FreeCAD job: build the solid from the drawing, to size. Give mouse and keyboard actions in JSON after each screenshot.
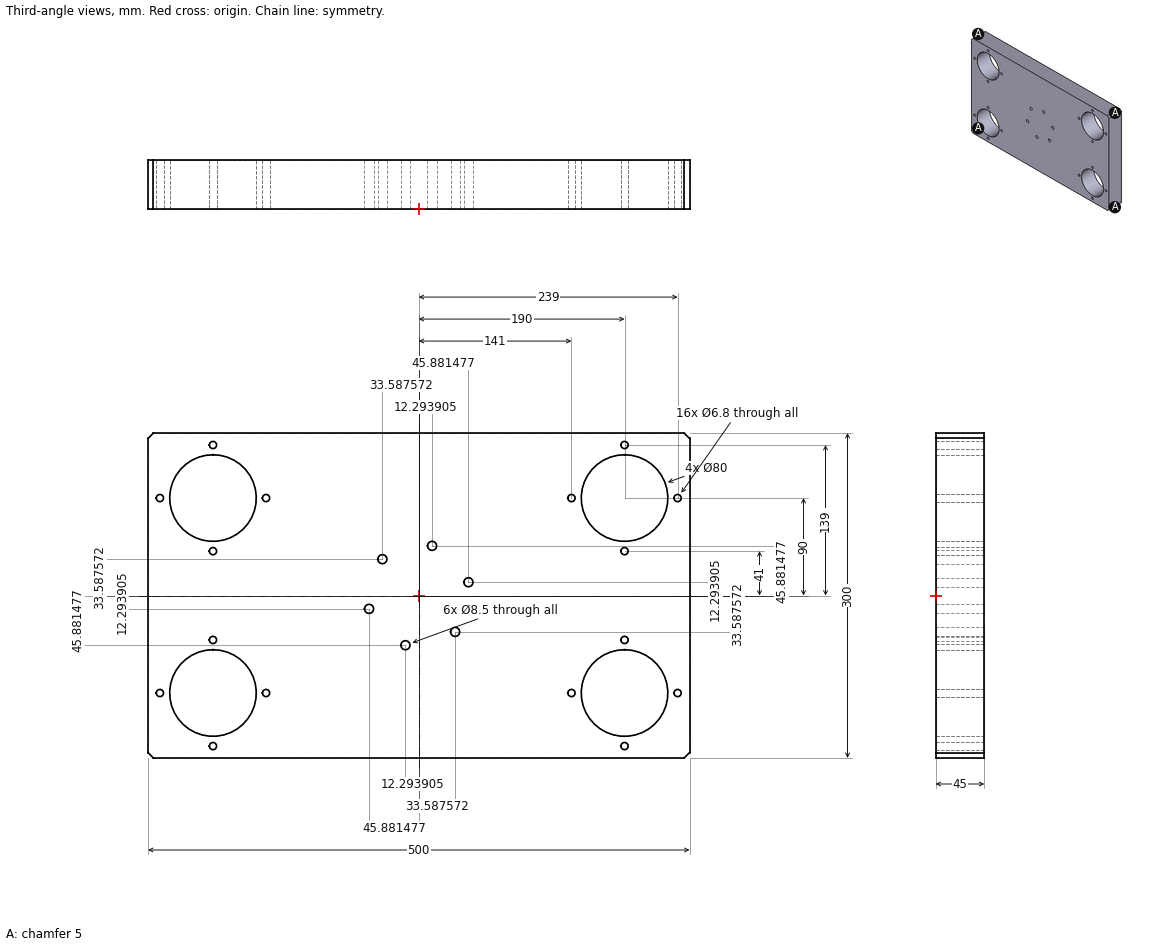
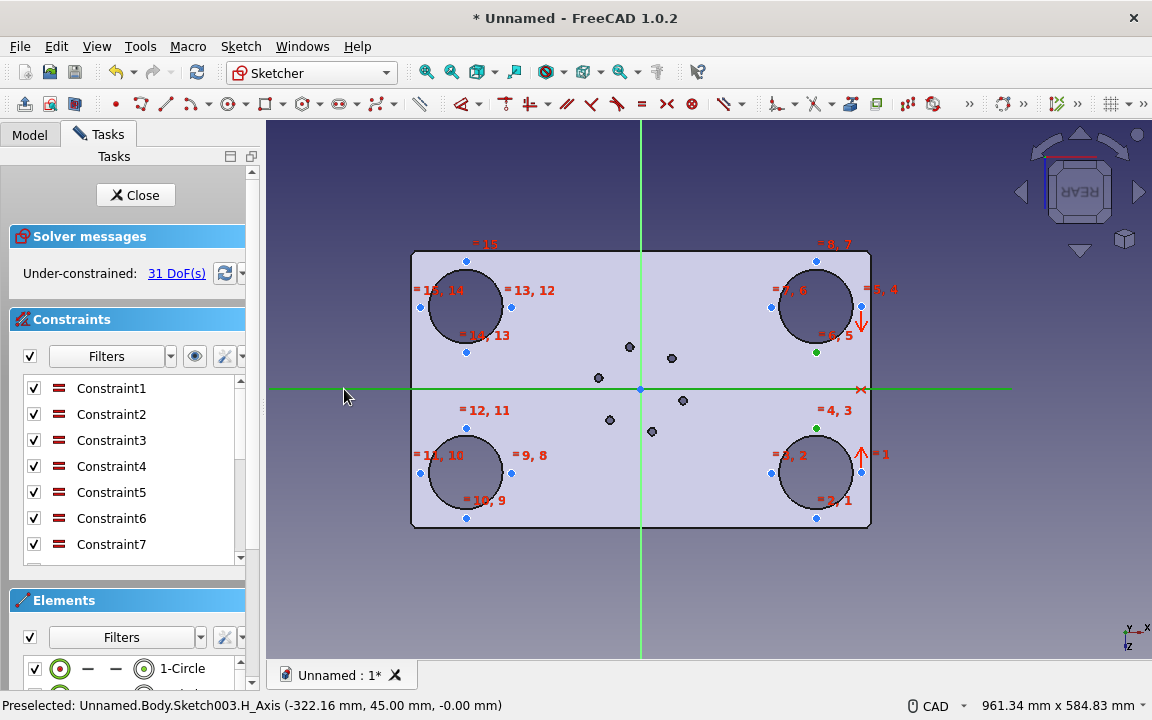
{"action": "left_click", "coordinate": [667, 104]}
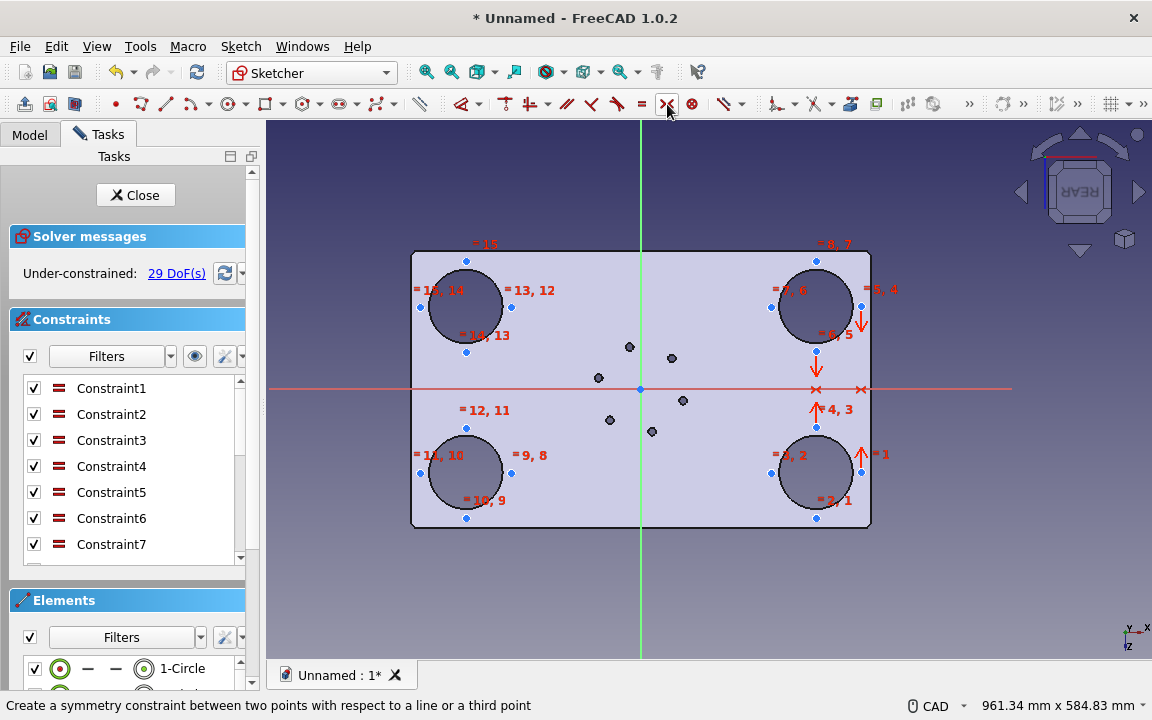
{"action": "left_click", "coordinate": [771, 473]}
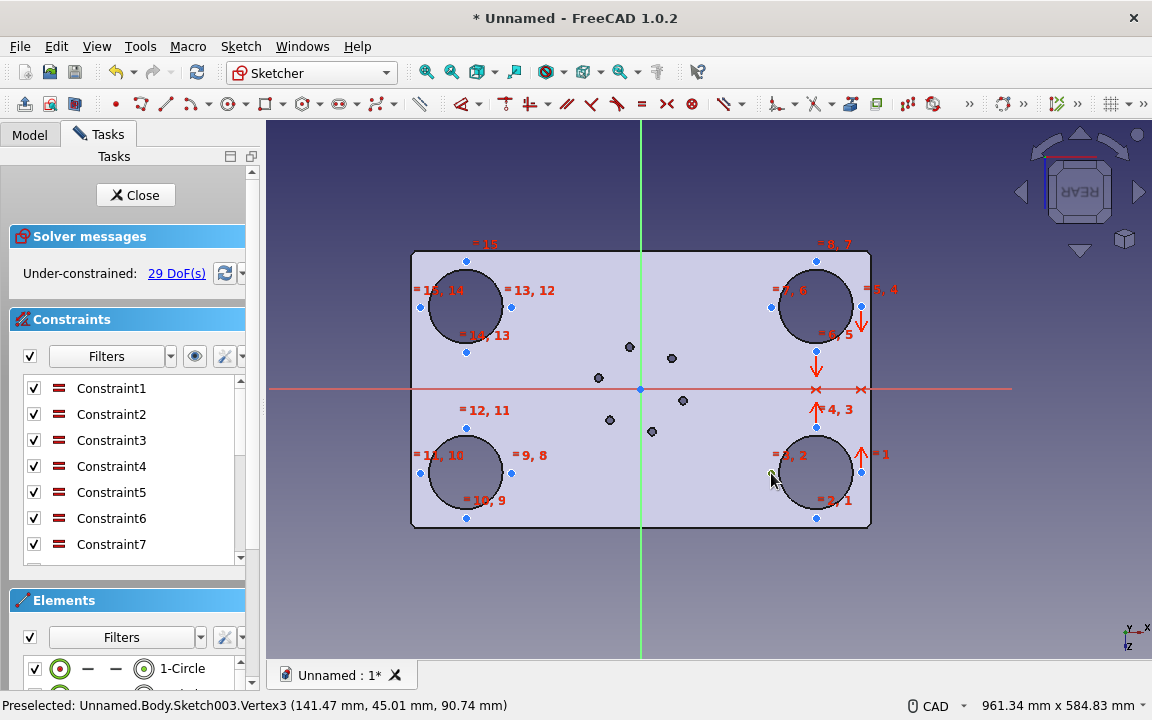
{"action": "left_click", "coordinate": [771, 308]}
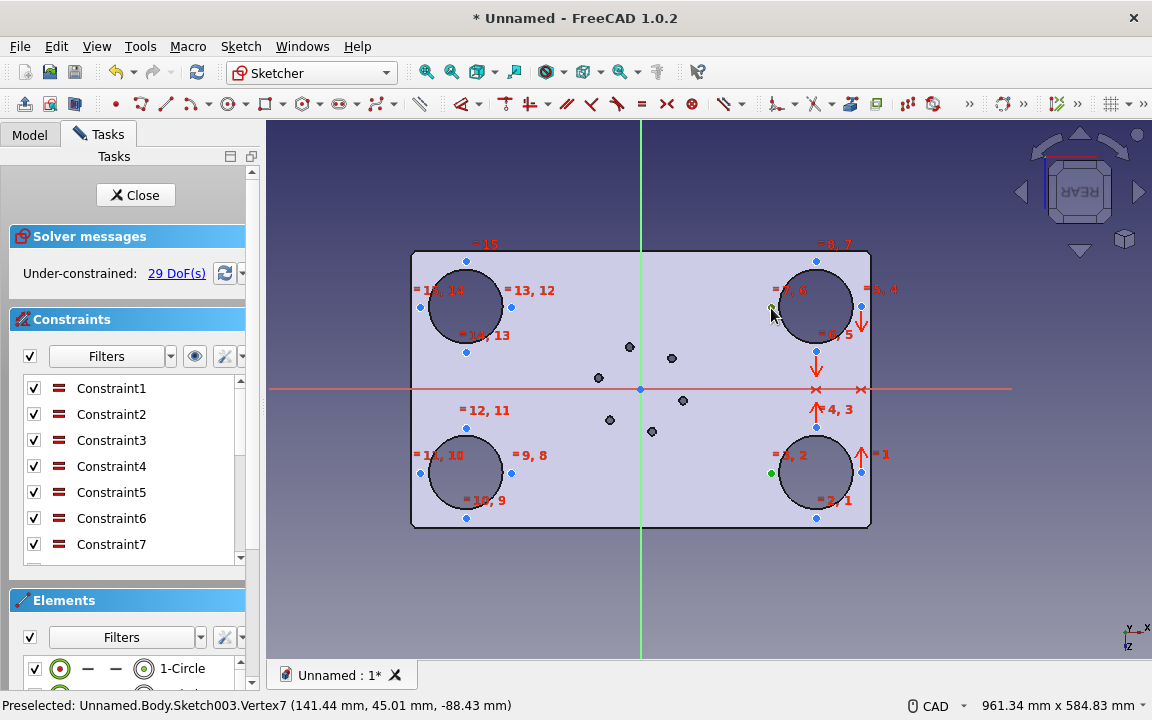
{"action": "left_click", "coordinate": [344, 389]}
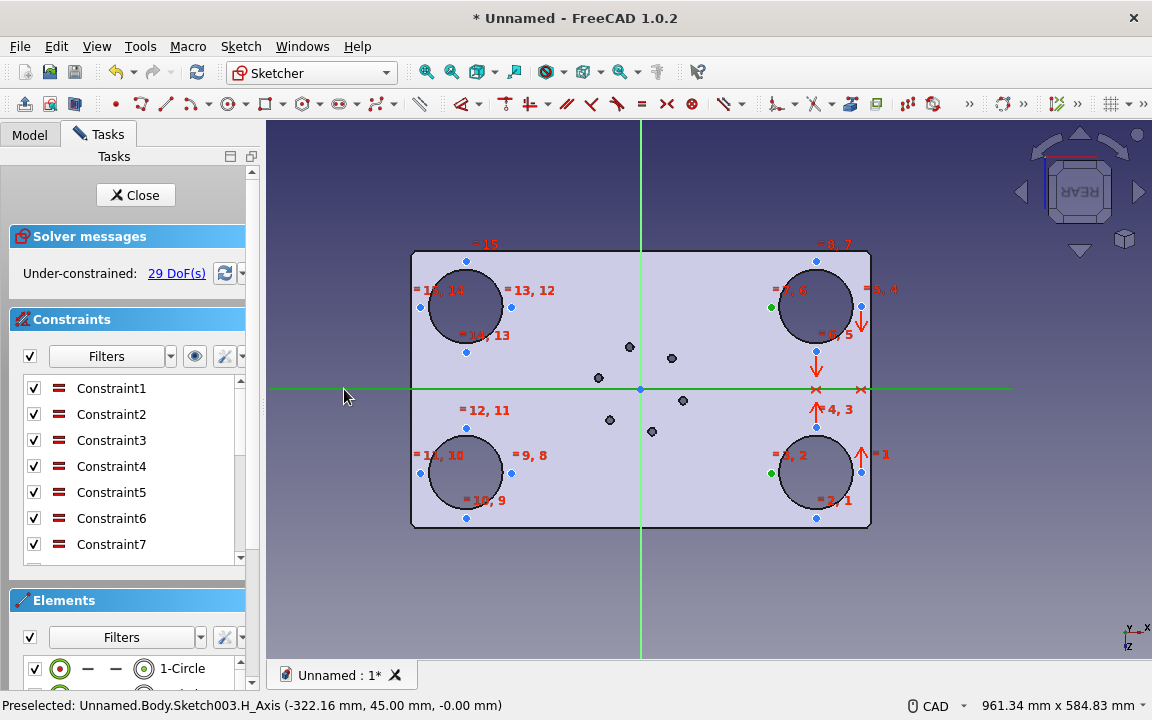
{"action": "left_click", "coordinate": [667, 104]}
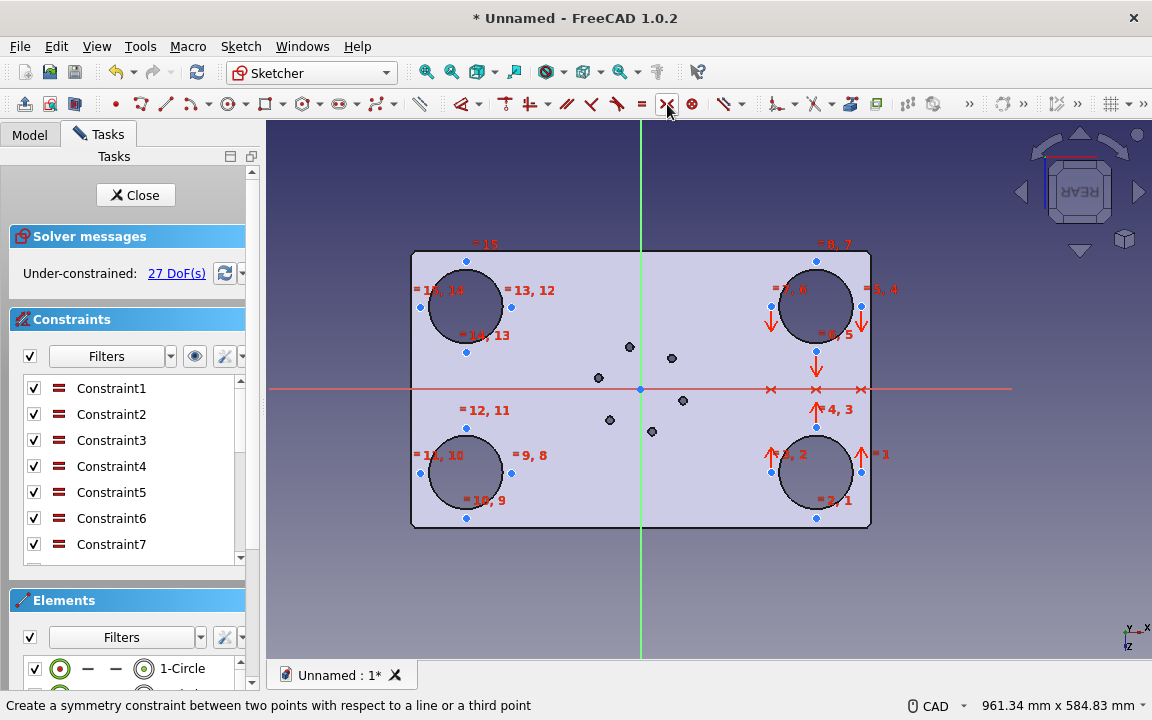
{"action": "left_click", "coordinate": [816, 518]}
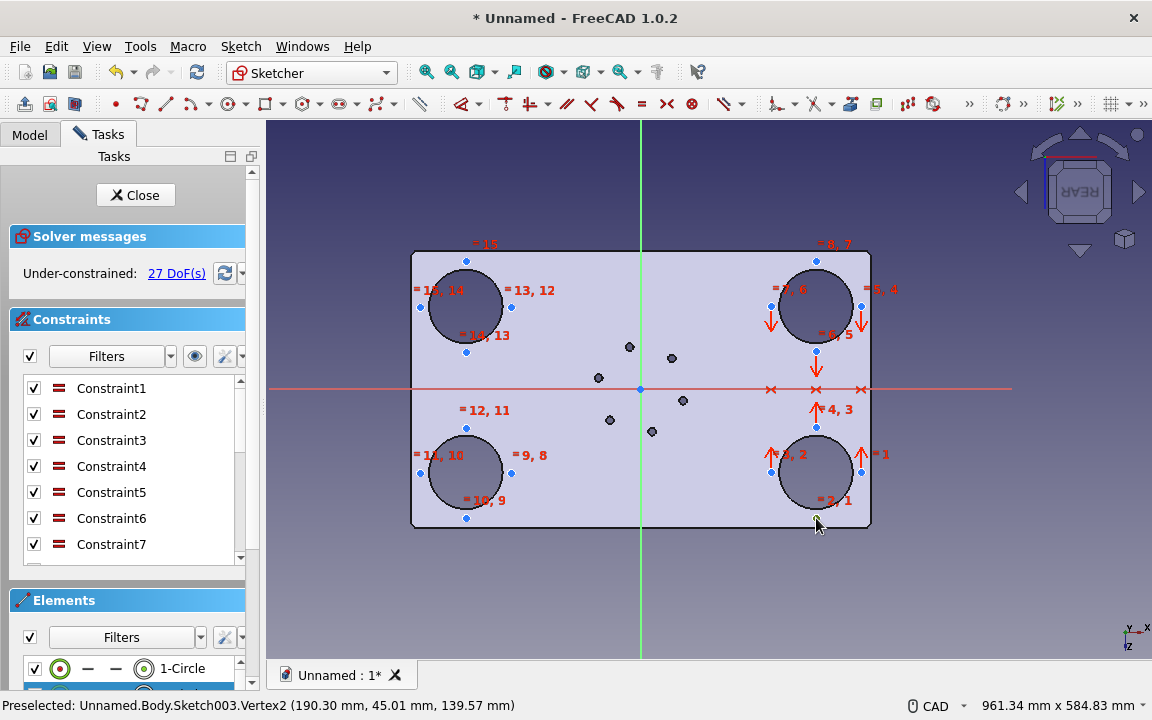
{"action": "left_click", "coordinate": [816, 262]}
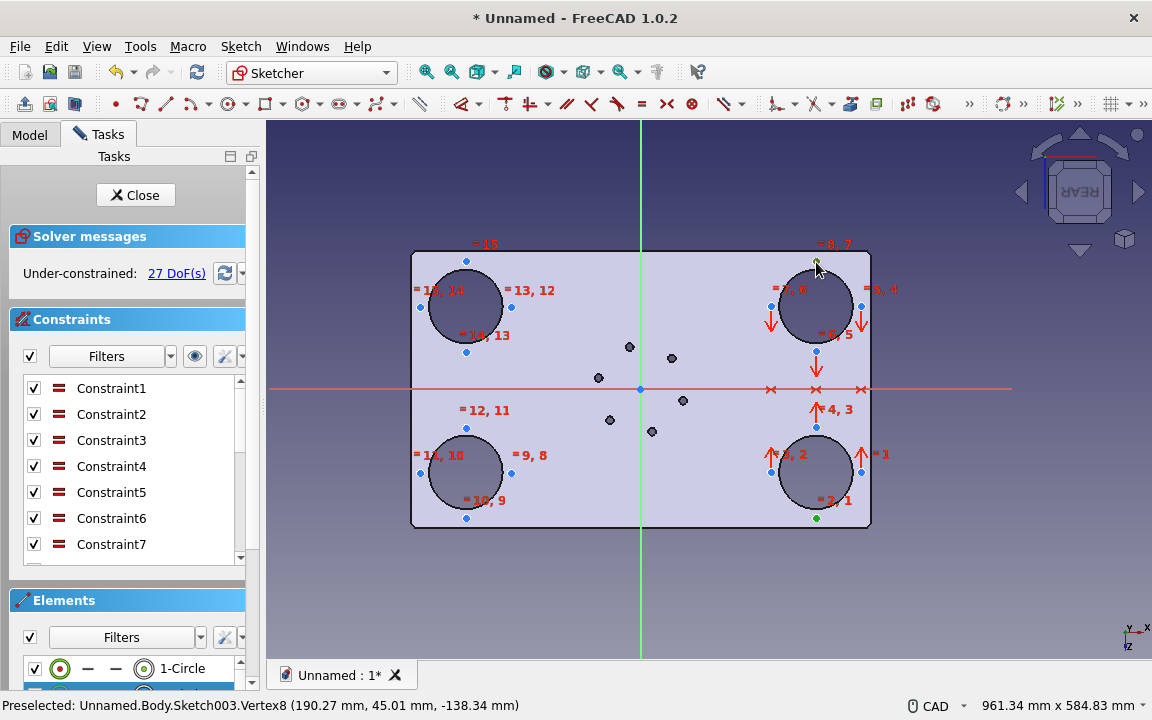
{"action": "left_click", "coordinate": [344, 389]}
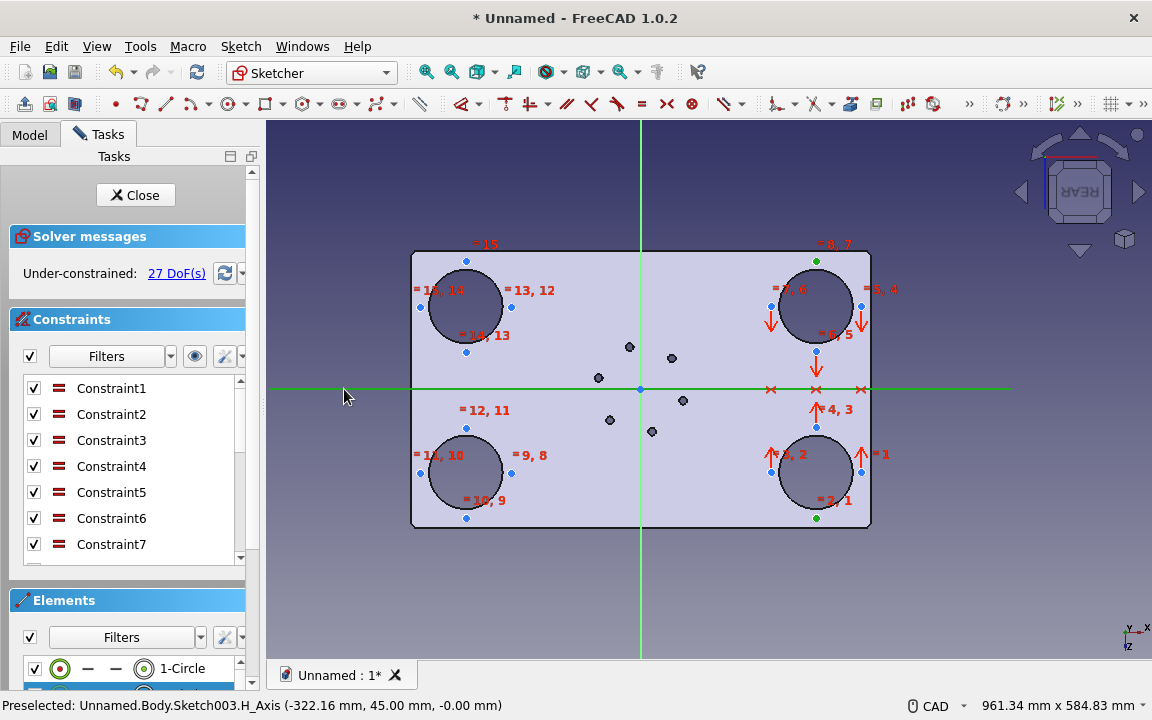
{"action": "left_click", "coordinate": [667, 104]}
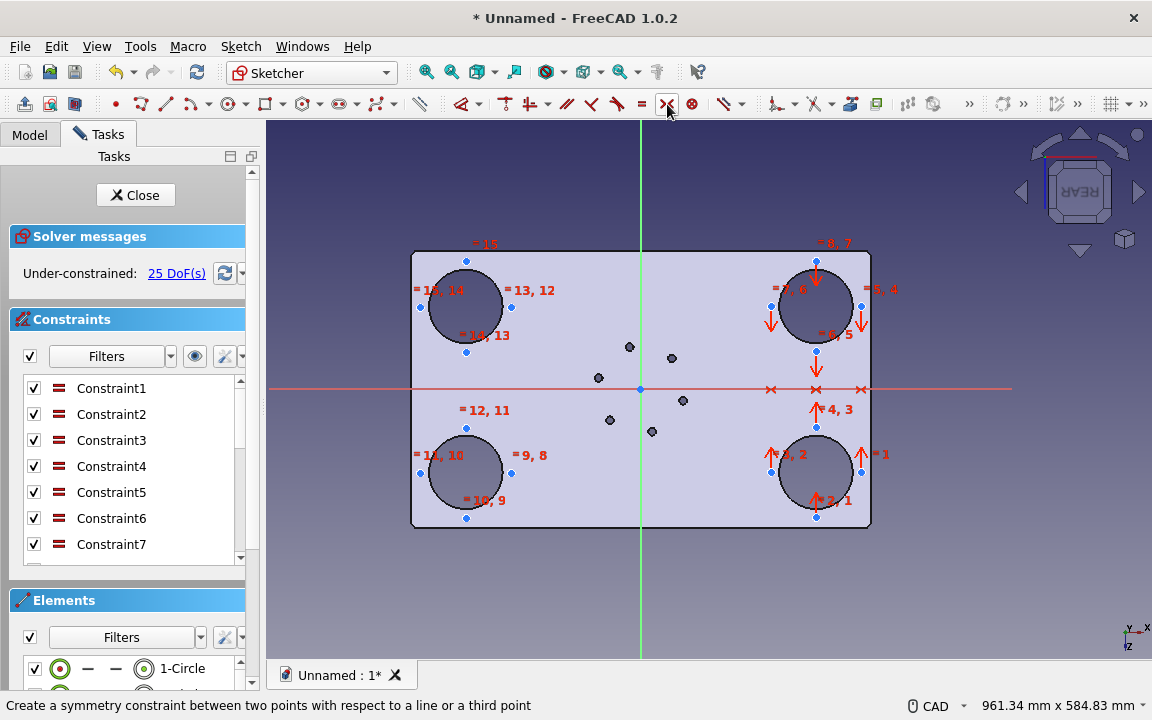
{"action": "left_click", "coordinate": [771, 472]}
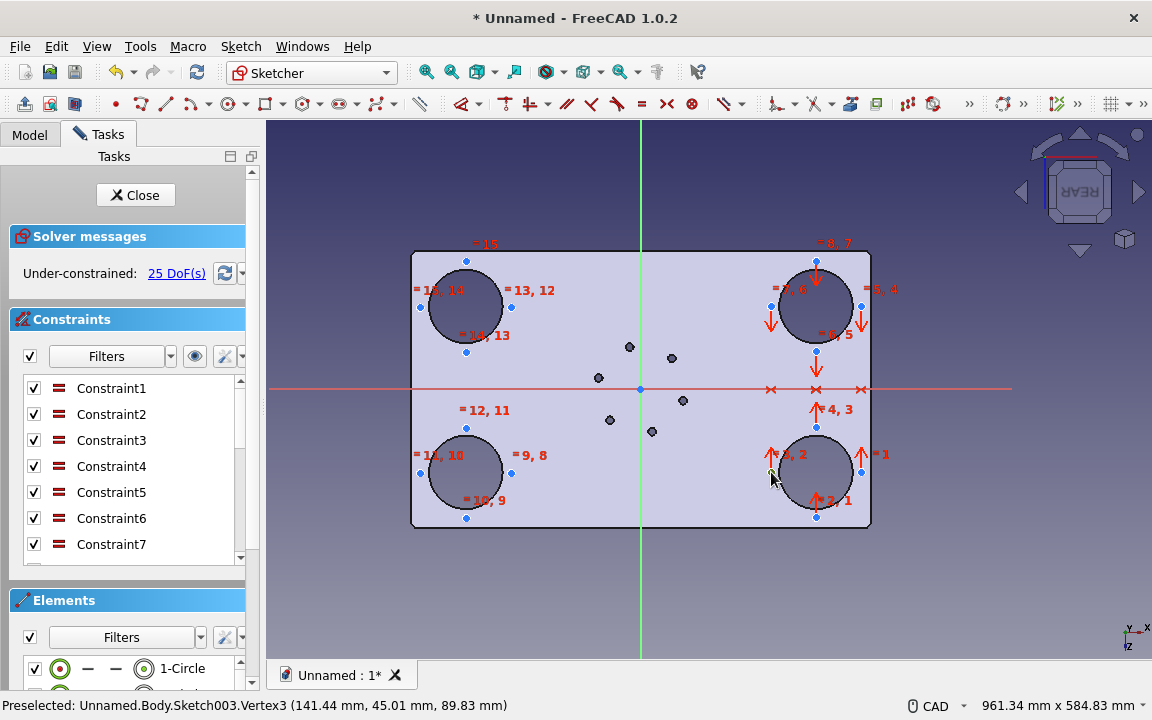
{"action": "left_click", "coordinate": [511, 473]}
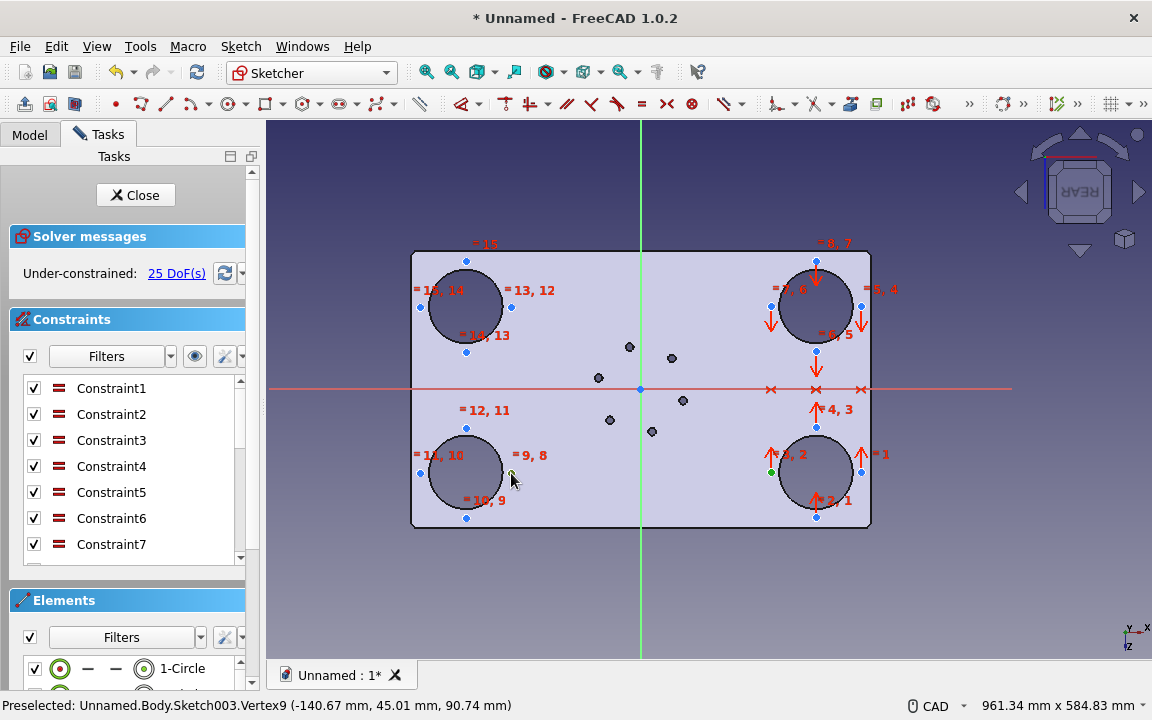
{"action": "left_click", "coordinate": [641, 596]}